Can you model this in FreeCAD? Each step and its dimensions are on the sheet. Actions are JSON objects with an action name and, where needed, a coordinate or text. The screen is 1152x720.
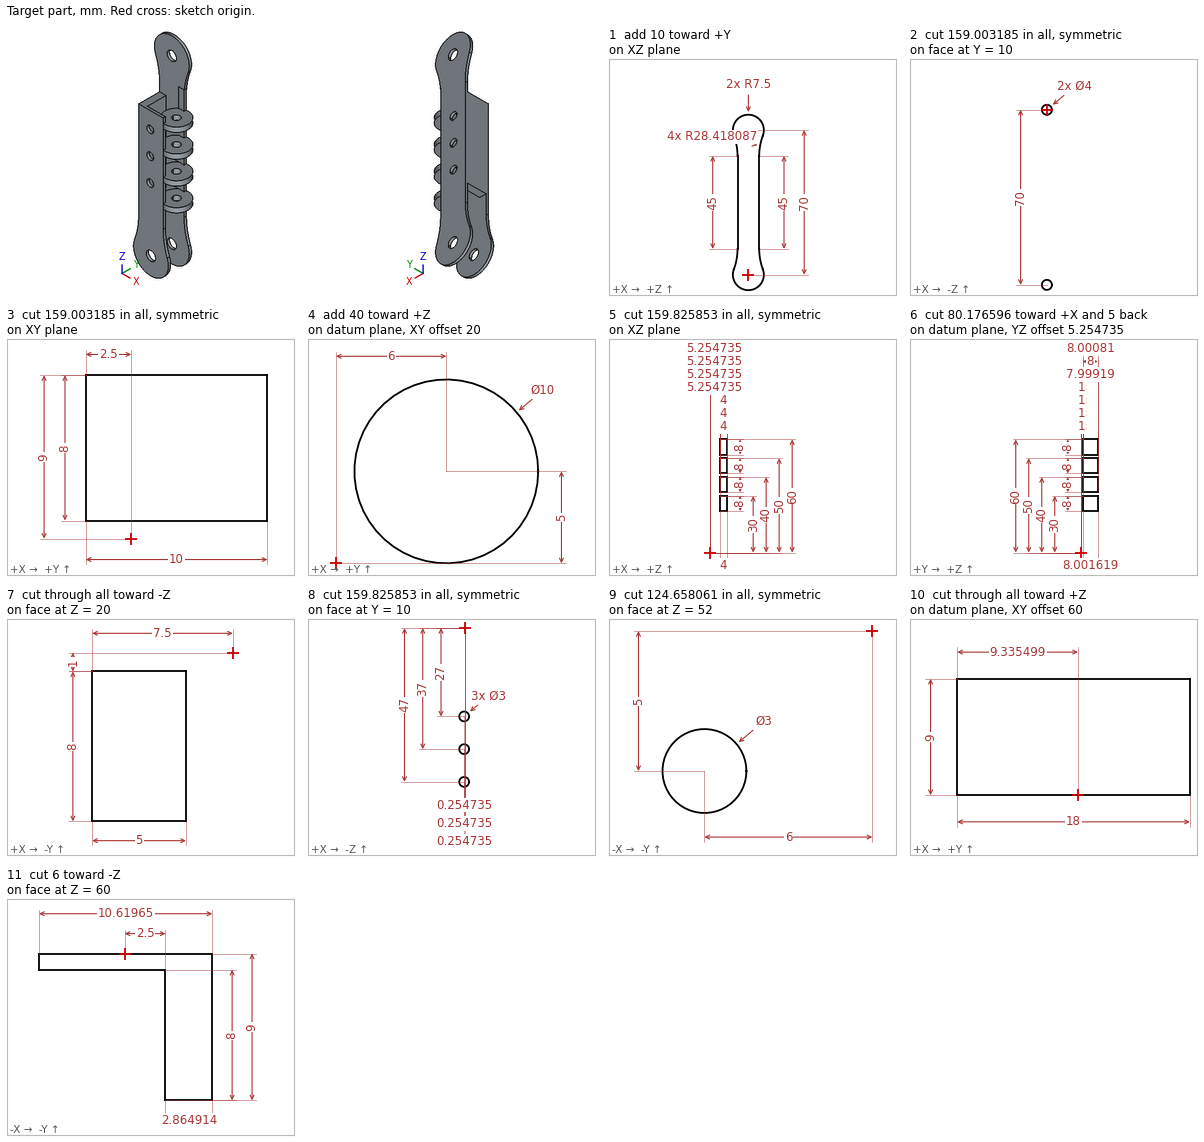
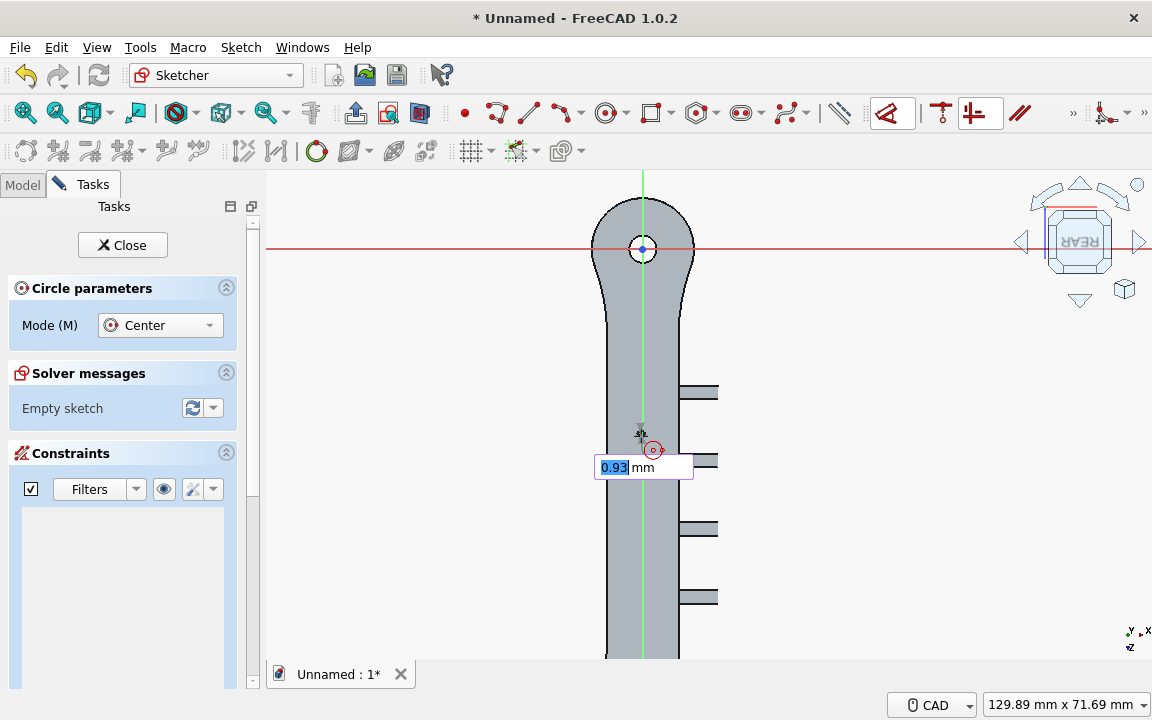
{"action": "scroll", "coordinate": [648, 426], "scroll_direction": "up", "scroll_amount": 6}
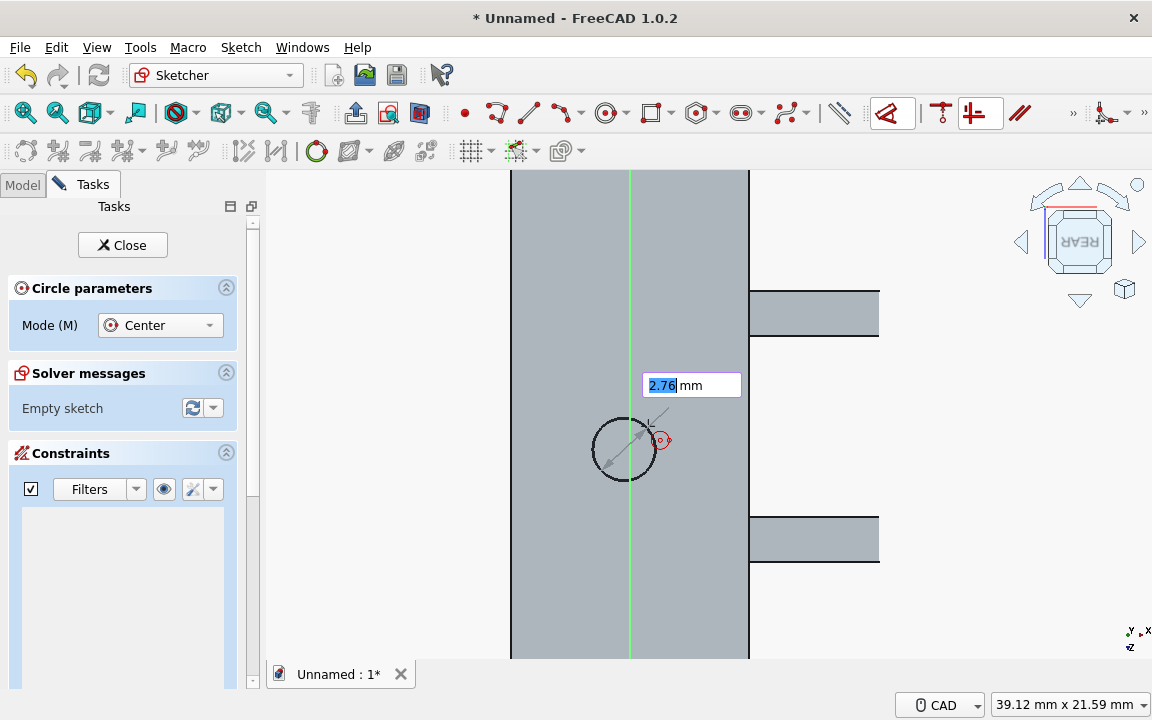
{"action": "left_click", "coordinate": [648, 425]}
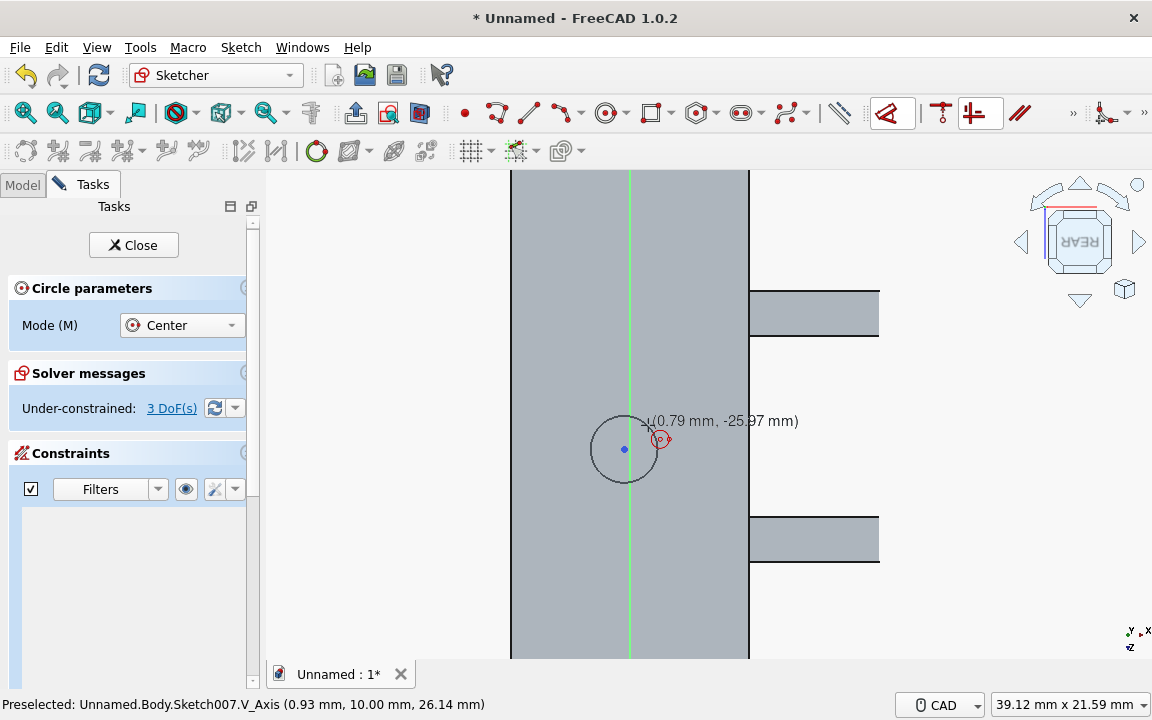
{"action": "scroll", "coordinate": [647, 426], "scroll_direction": "down", "scroll_amount": 6}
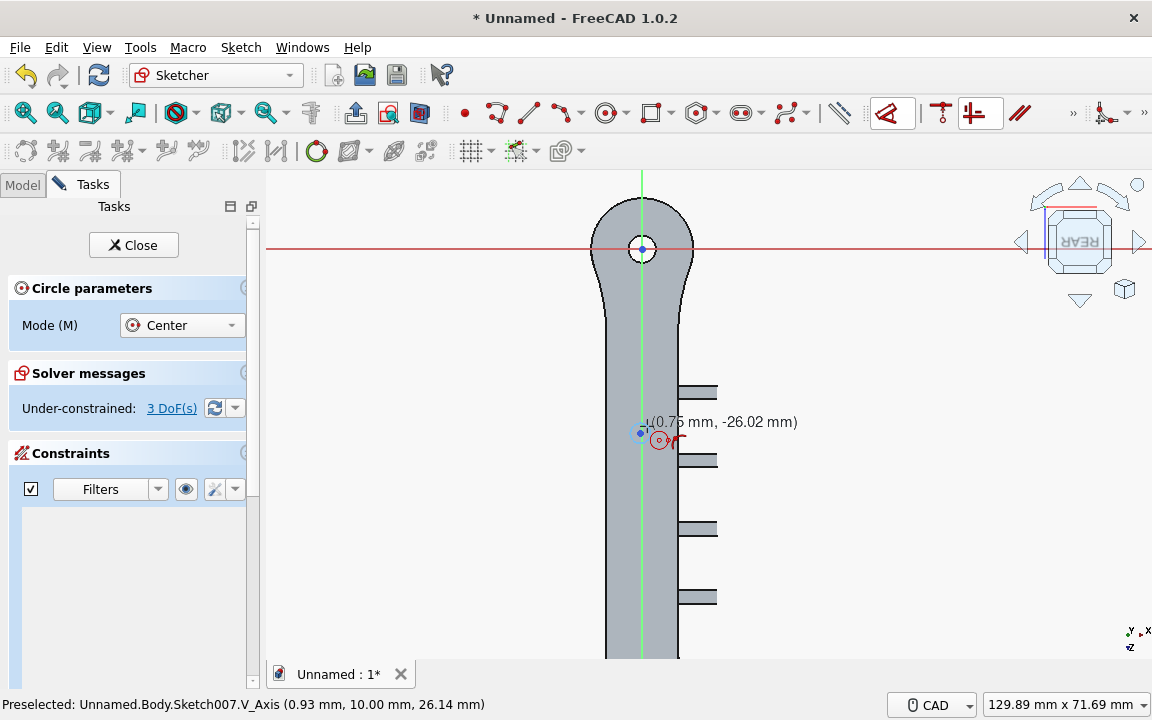
{"action": "scroll", "coordinate": [640, 502], "scroll_direction": "up", "scroll_amount": 12}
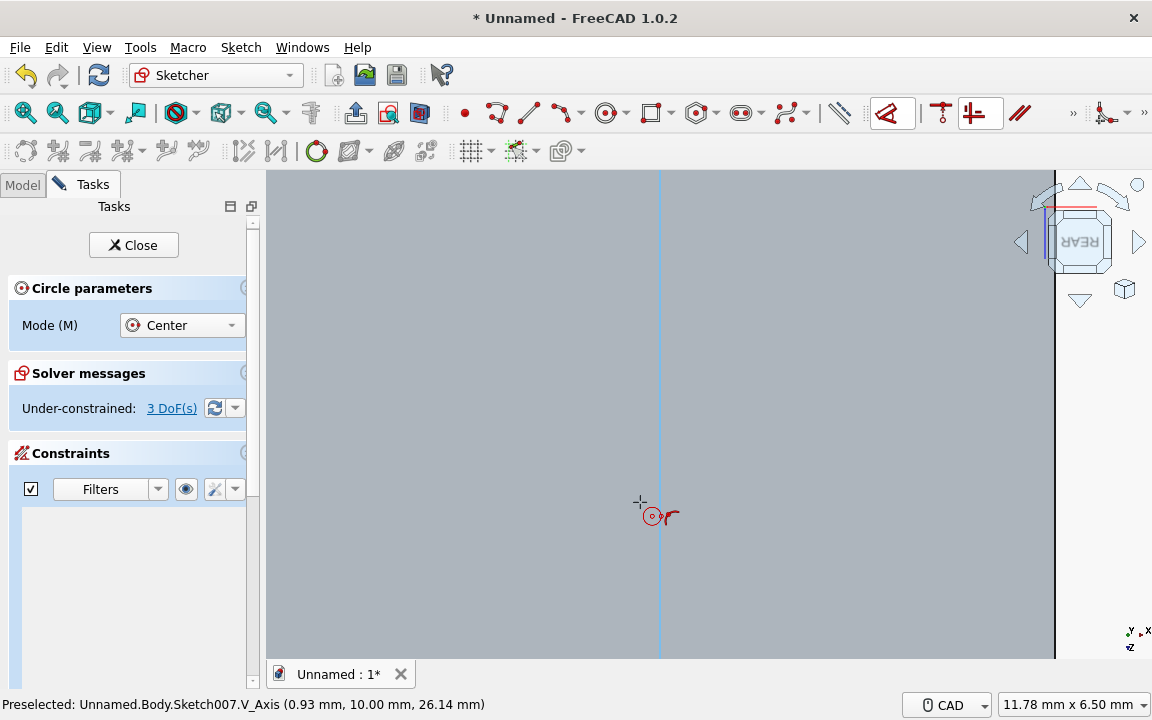
{"action": "left_click", "coordinate": [641, 490]}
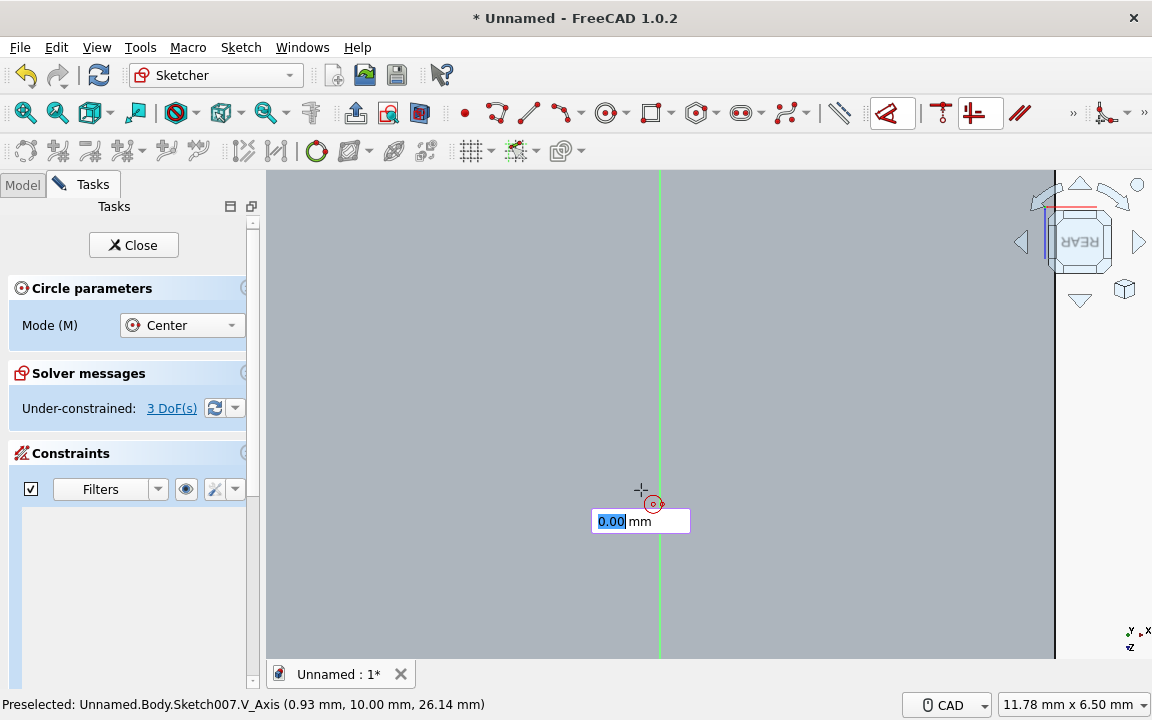
{"action": "scroll", "coordinate": [640, 503], "scroll_direction": "down", "scroll_amount": 12}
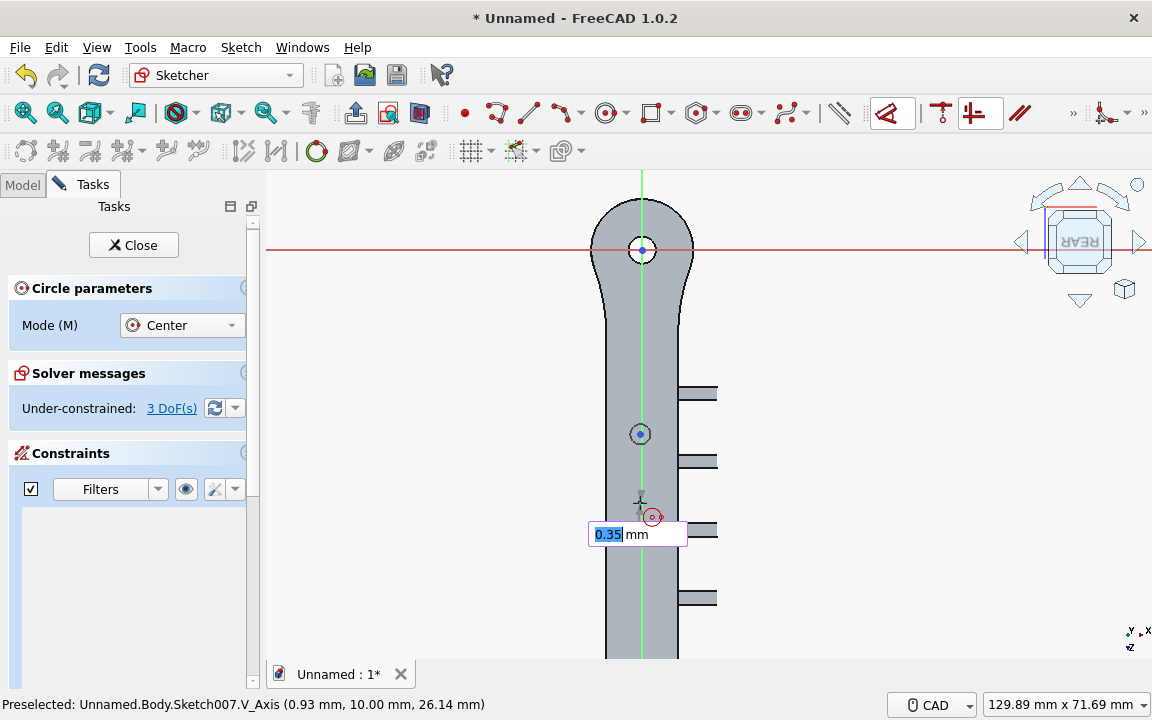
{"action": "scroll", "coordinate": [648, 495], "scroll_direction": "up", "scroll_amount": 6}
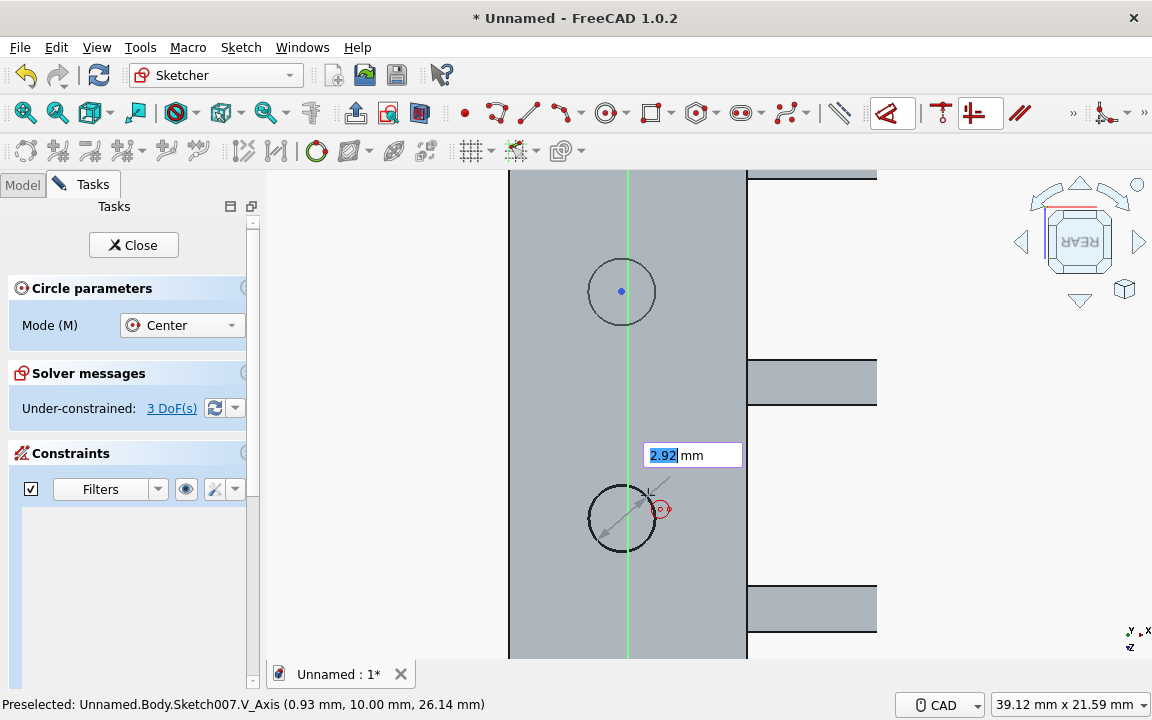
{"action": "left_click", "coordinate": [646, 494]}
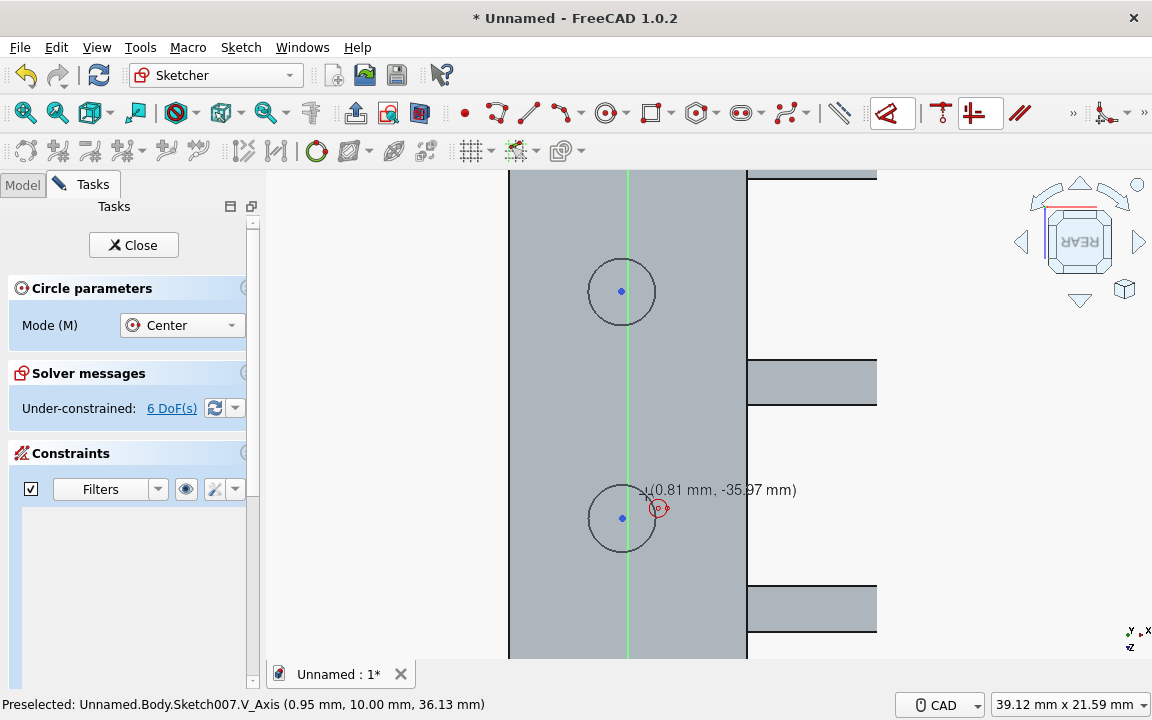
{"action": "scroll", "coordinate": [648, 494], "scroll_direction": "down", "scroll_amount": 6}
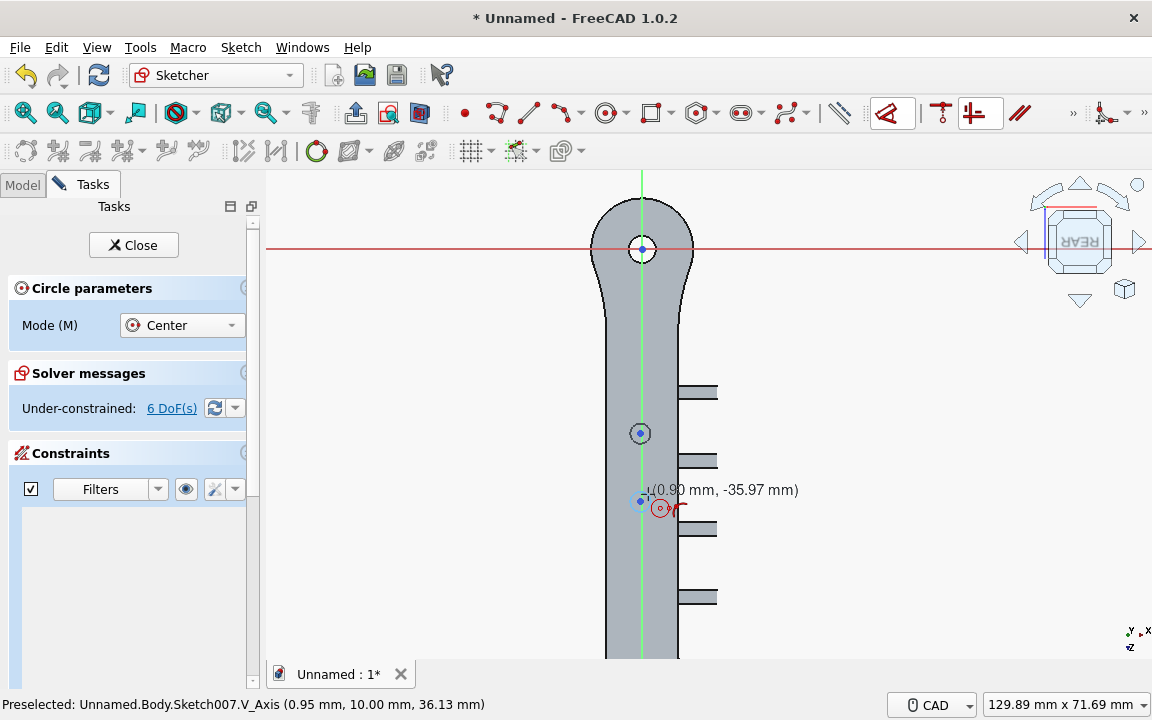
{"action": "scroll", "coordinate": [640, 570], "scroll_direction": "up", "scroll_amount": 12}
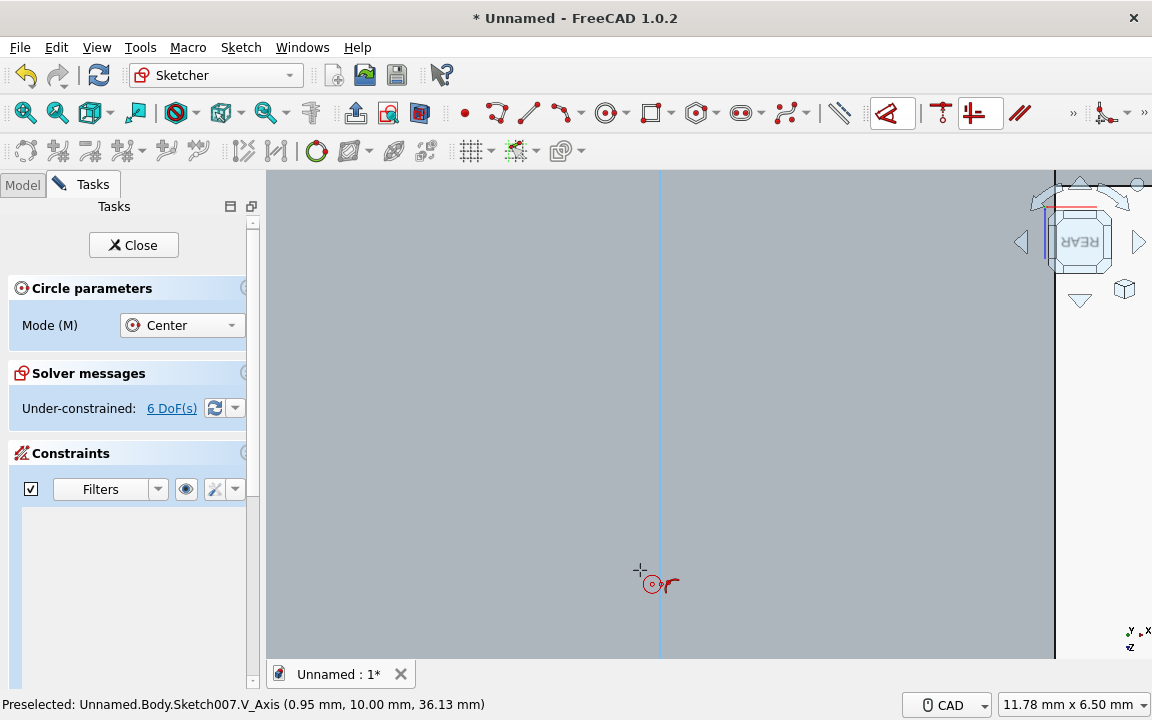
{"action": "left_click", "coordinate": [641, 562]}